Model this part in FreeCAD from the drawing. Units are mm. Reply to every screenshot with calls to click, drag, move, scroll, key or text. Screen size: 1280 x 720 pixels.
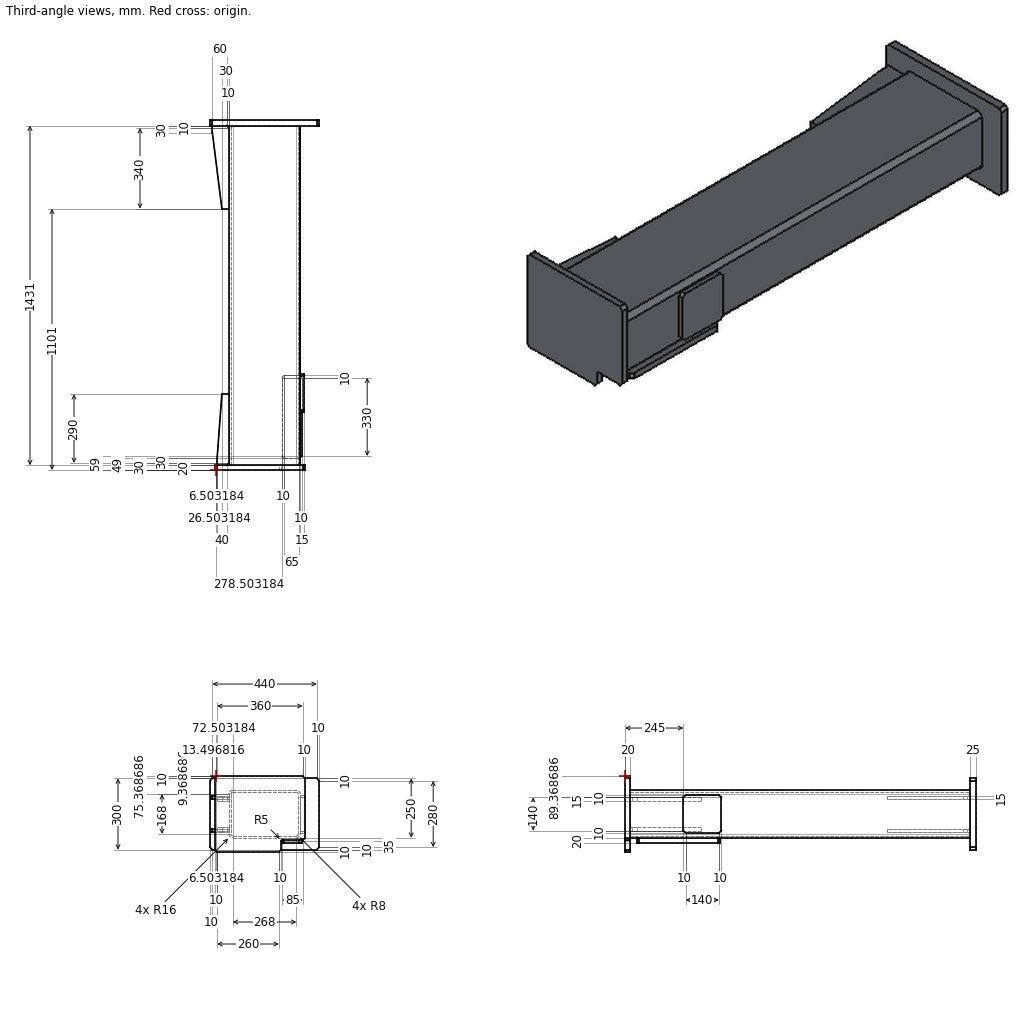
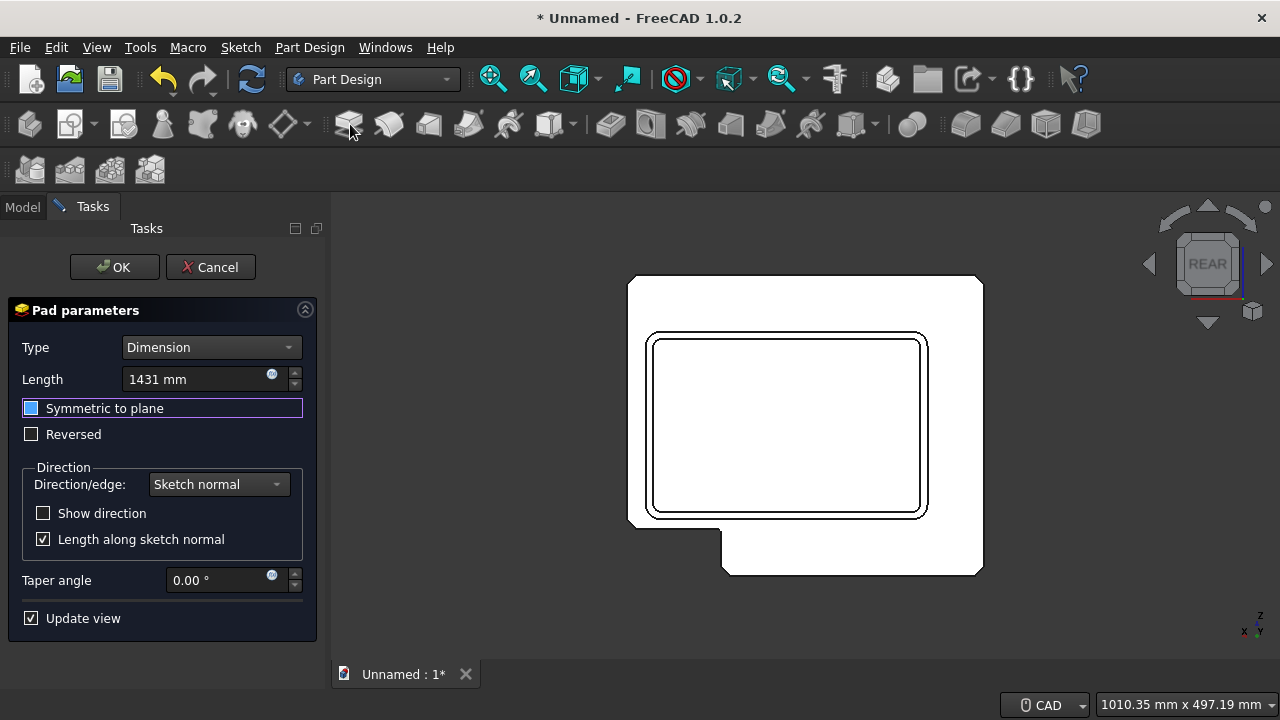
click(115, 267)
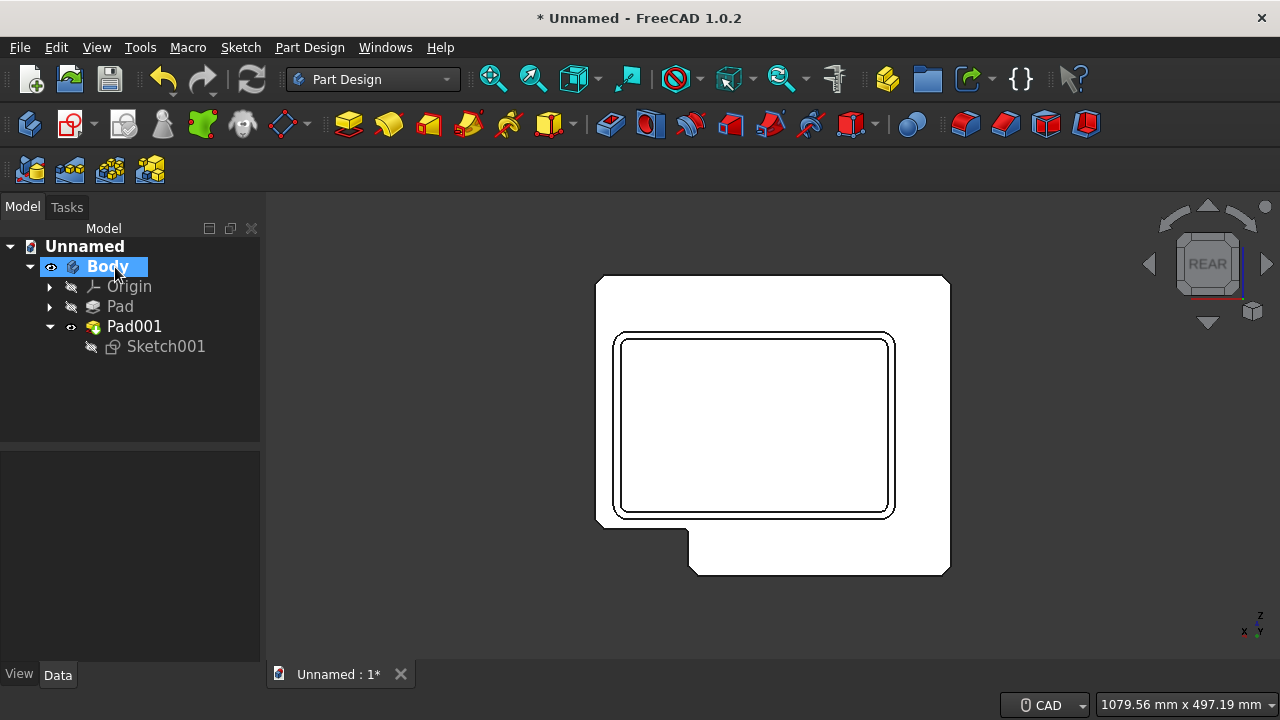
scroll(620, 336, up, 8)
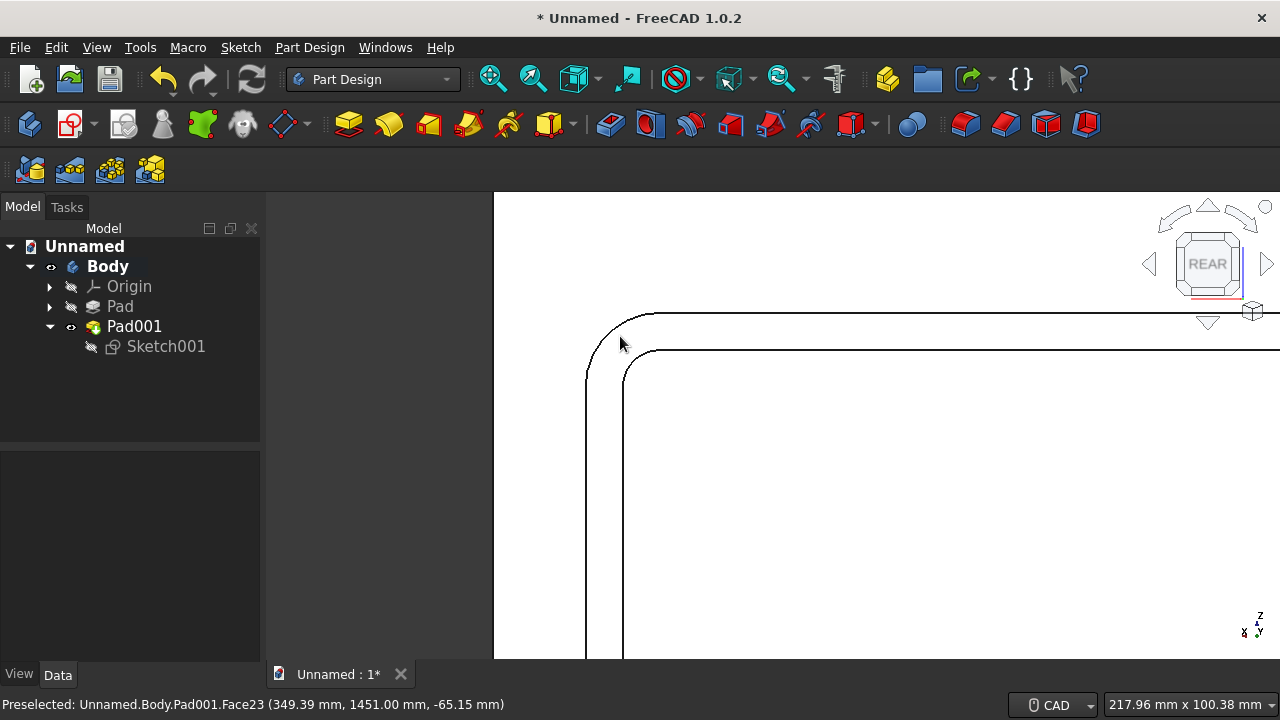
click(619, 340)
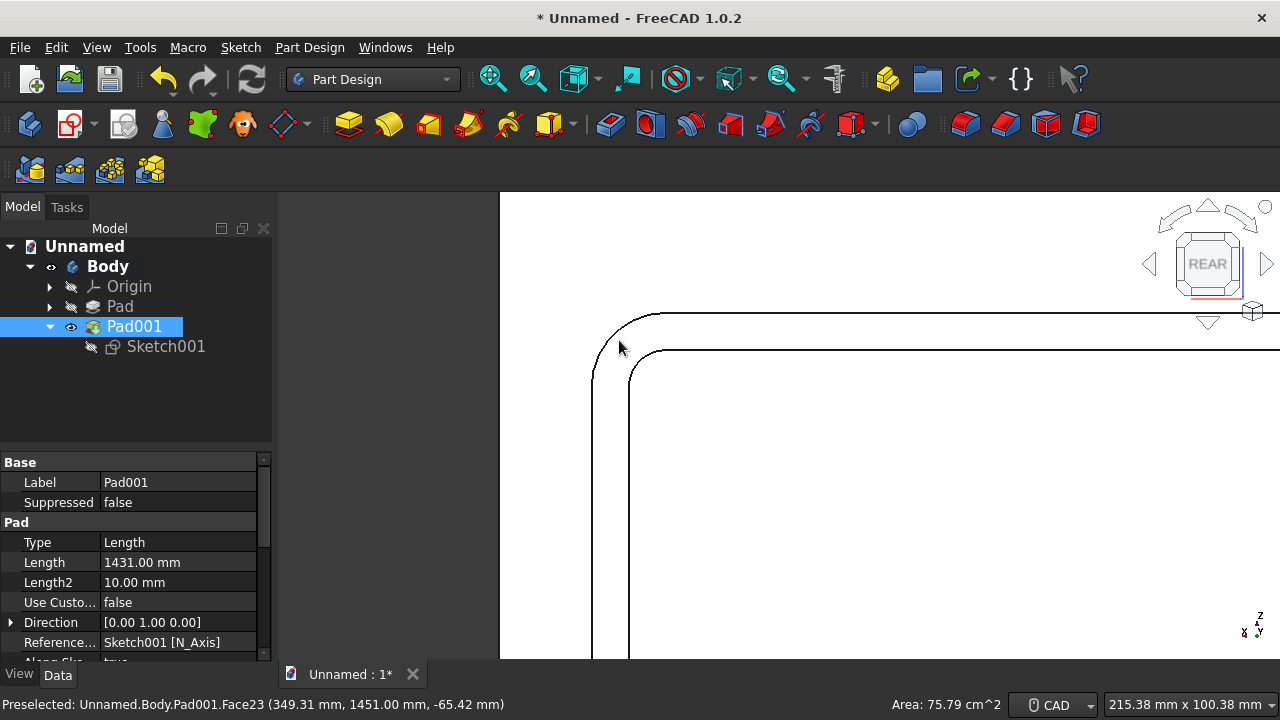
click(70, 124)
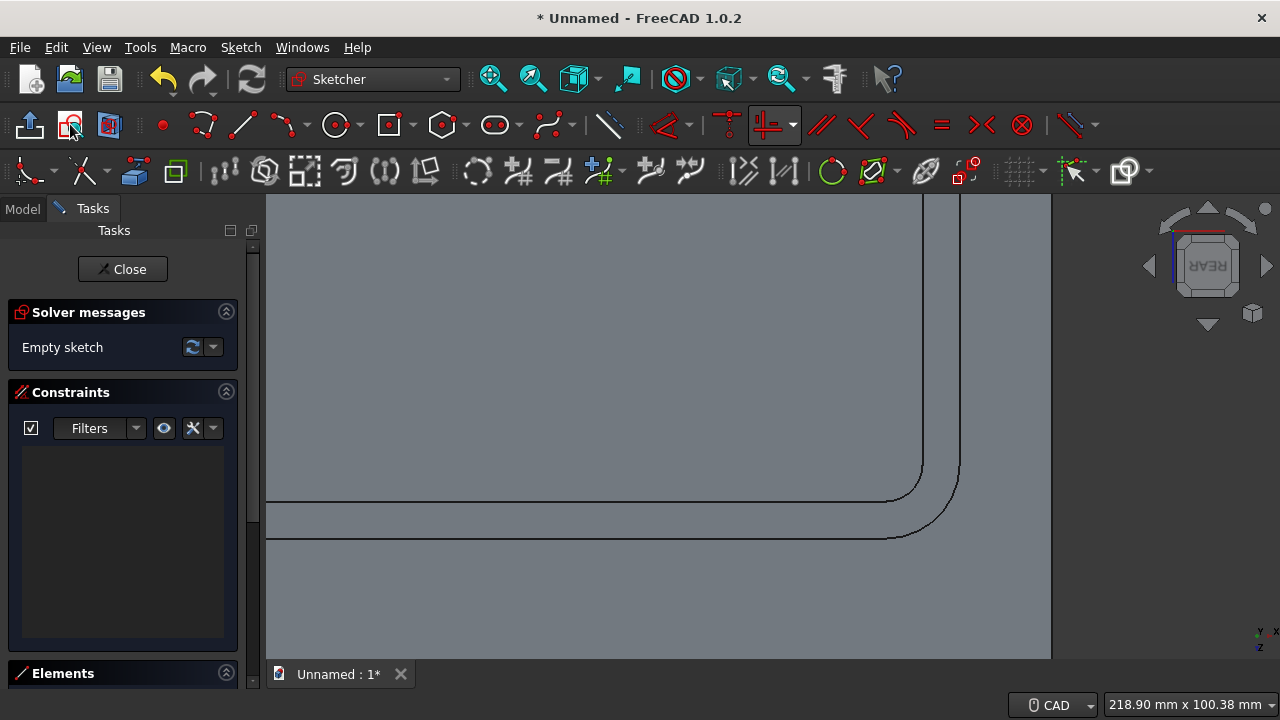
scroll(816, 510, down, 8)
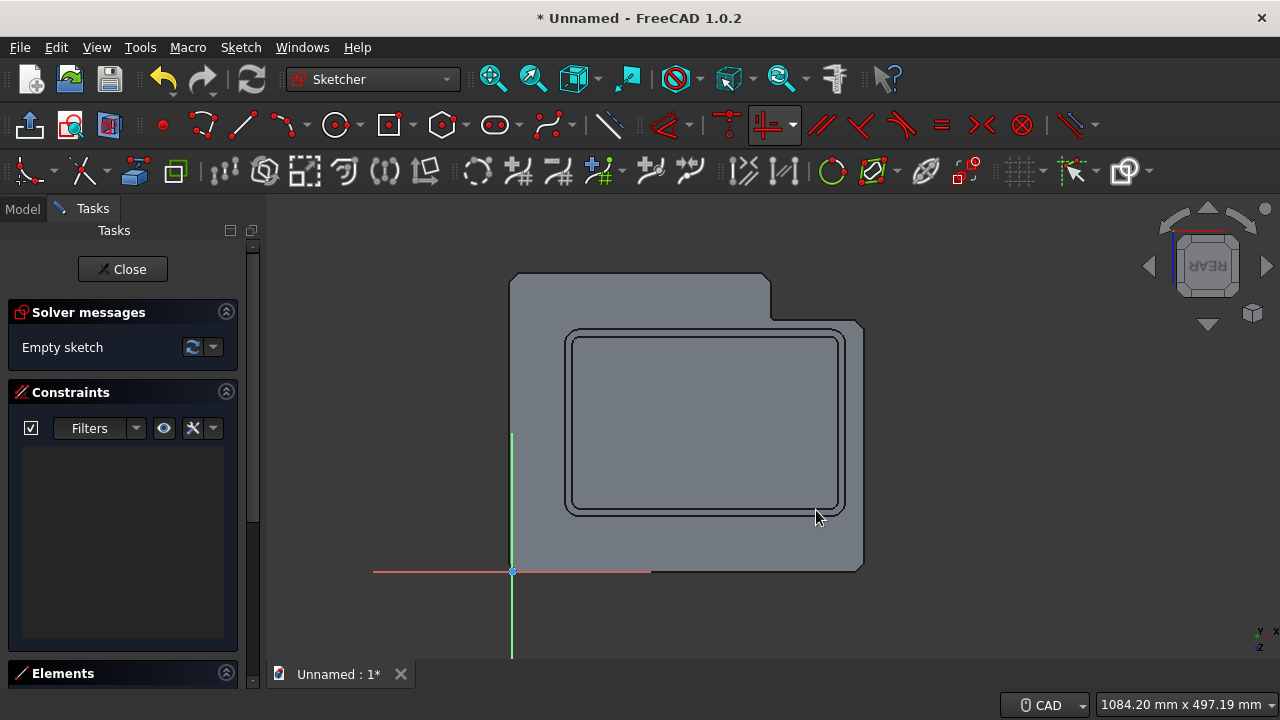
click(204, 126)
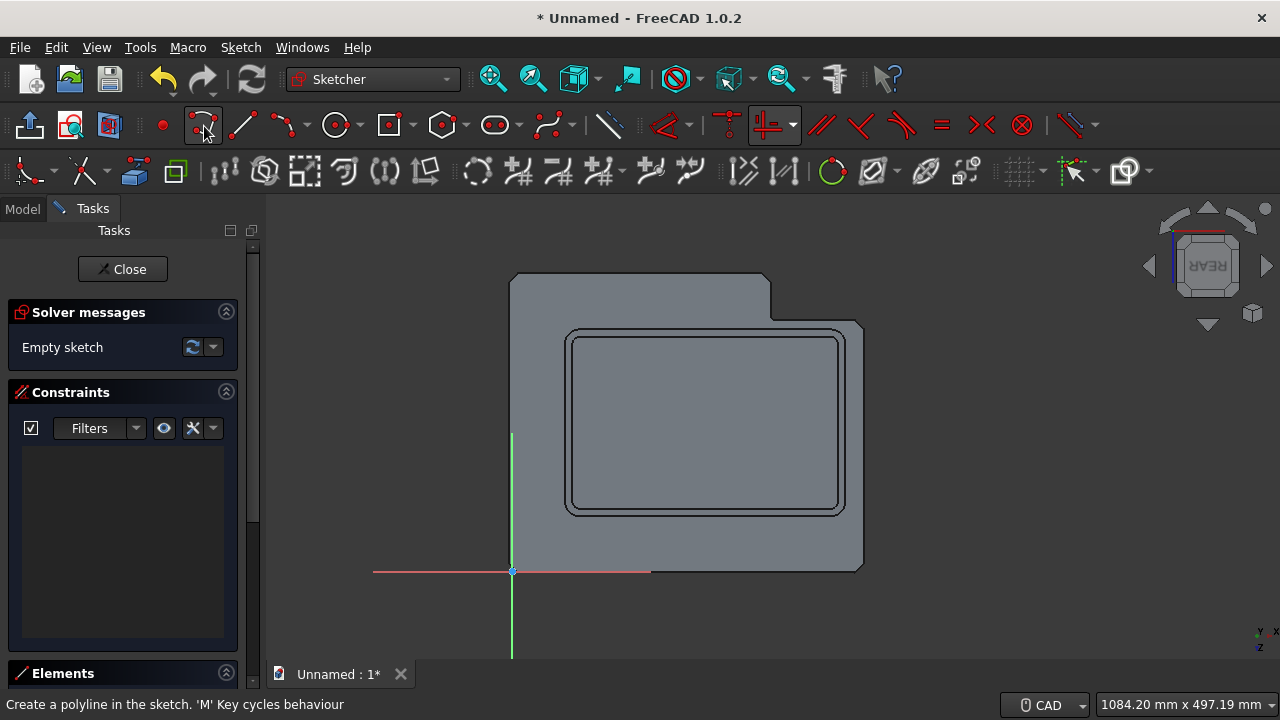
scroll(499, 563, up, 3)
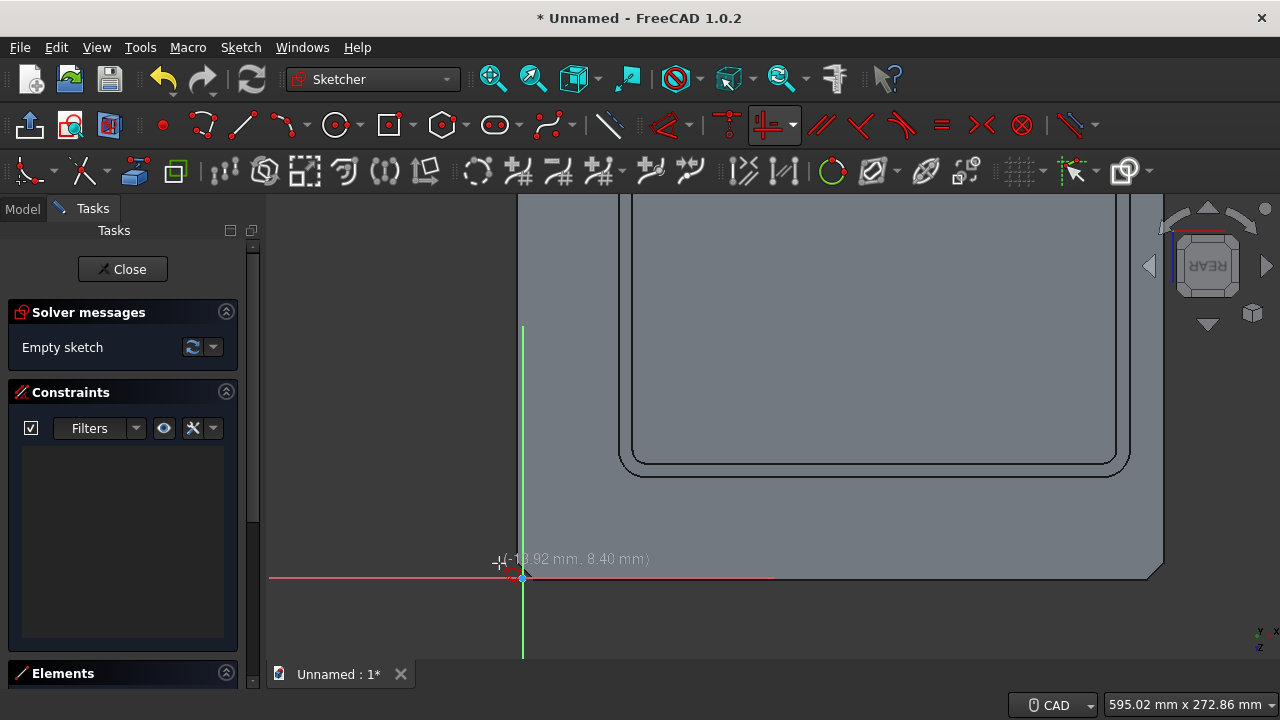
click(500, 563)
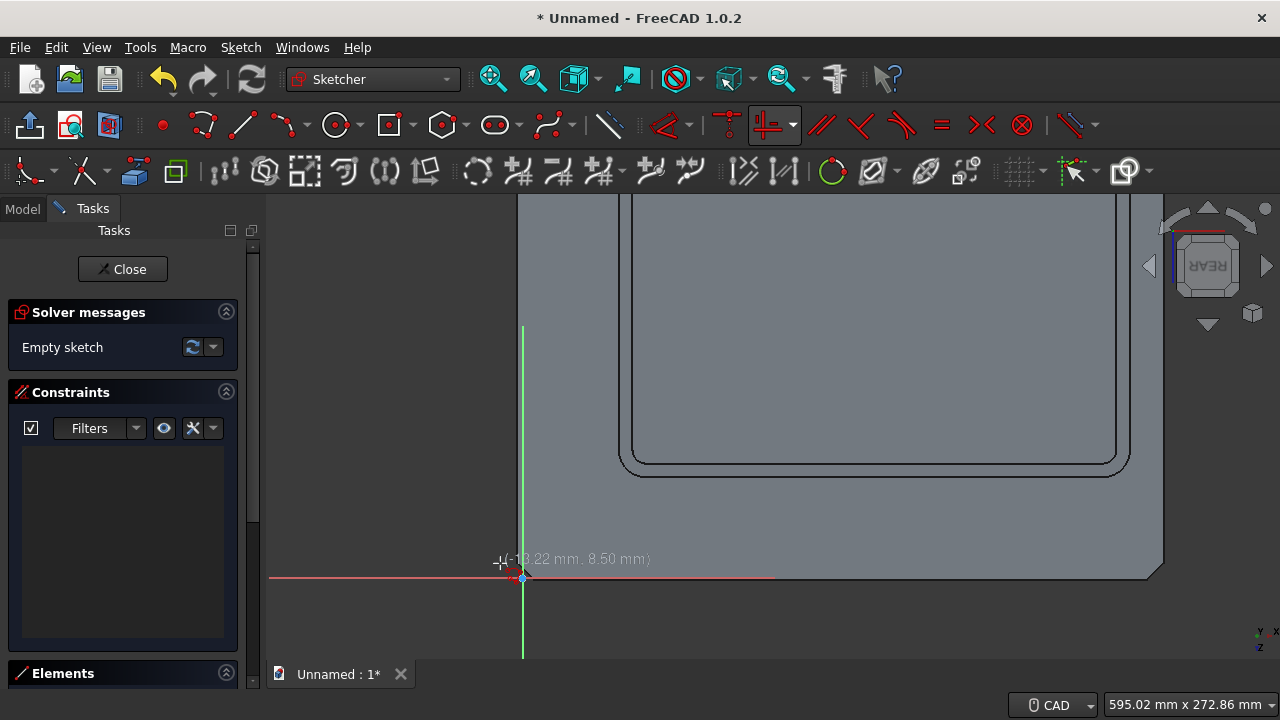
scroll(498, 562, down, 3)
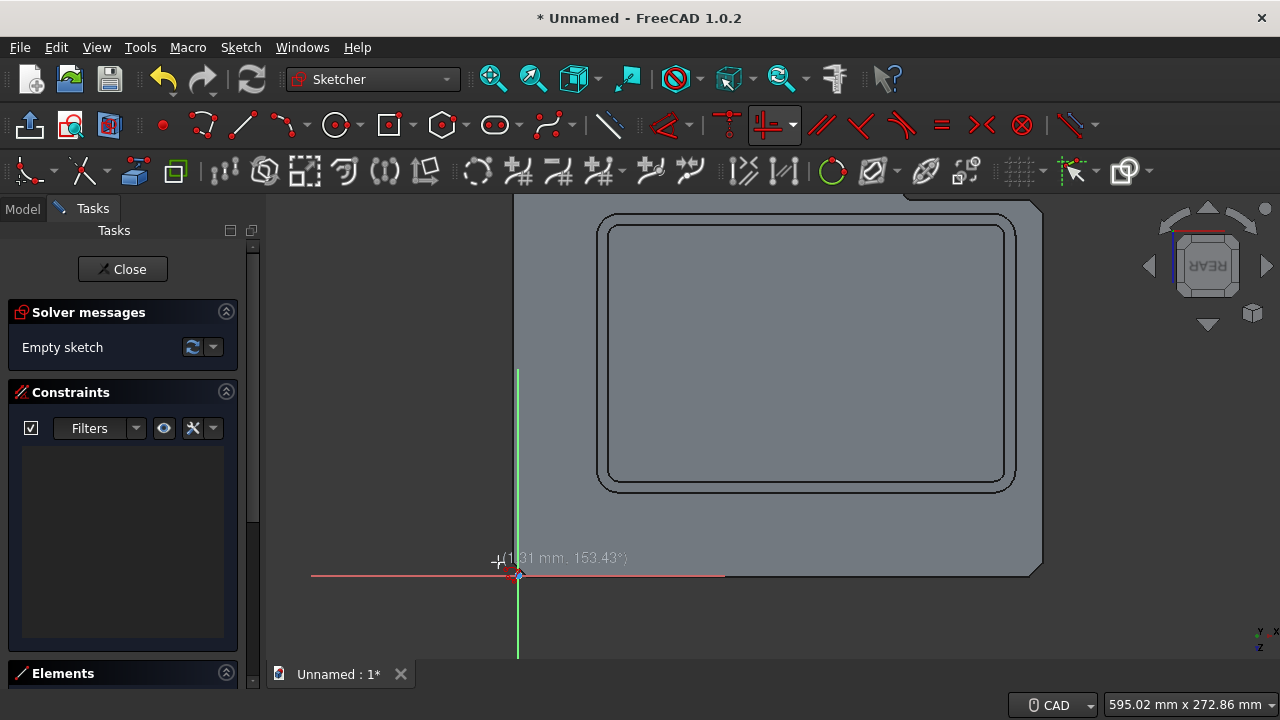
scroll(910, 563, up, 3)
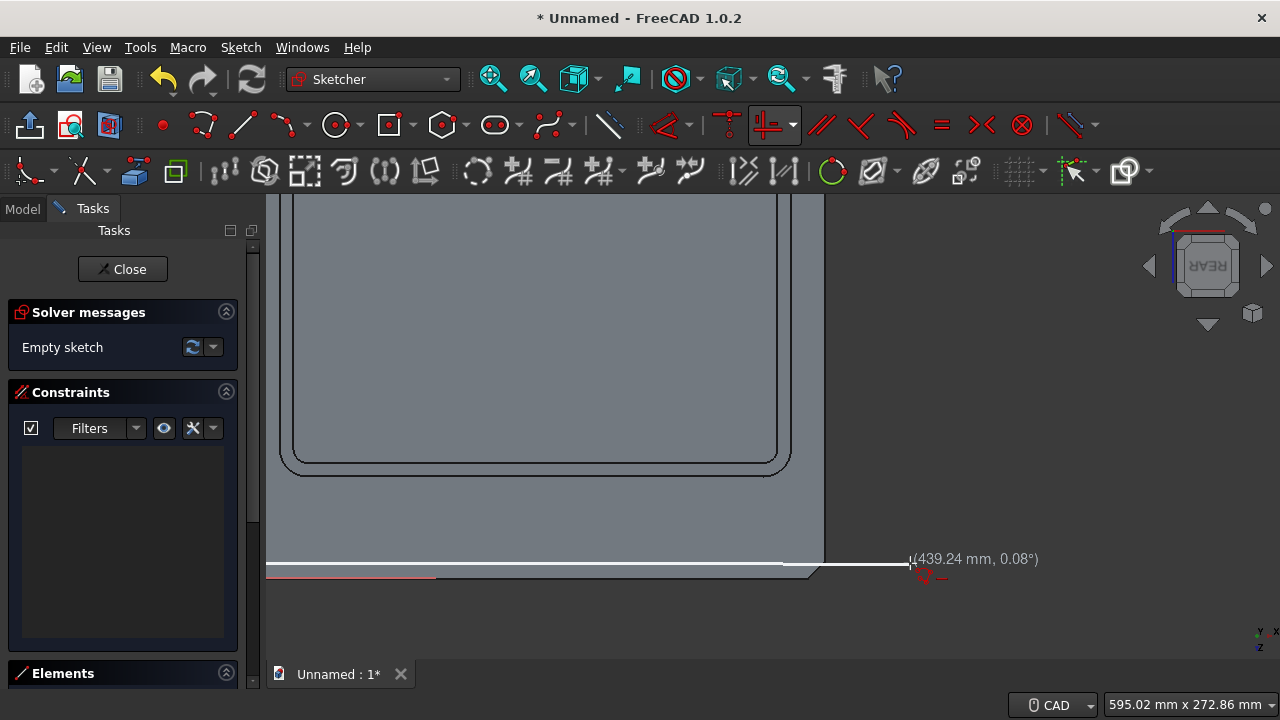
click(910, 562)
click(927, 545)